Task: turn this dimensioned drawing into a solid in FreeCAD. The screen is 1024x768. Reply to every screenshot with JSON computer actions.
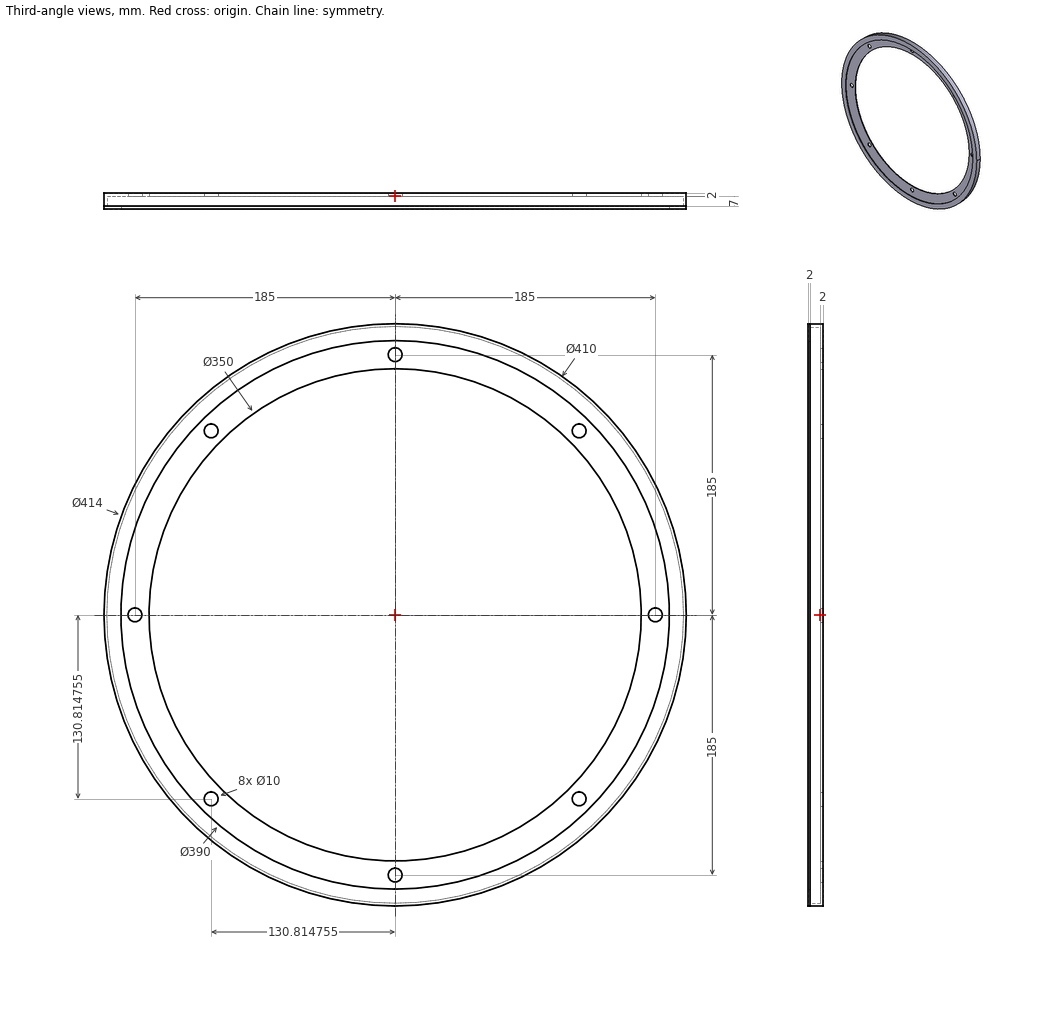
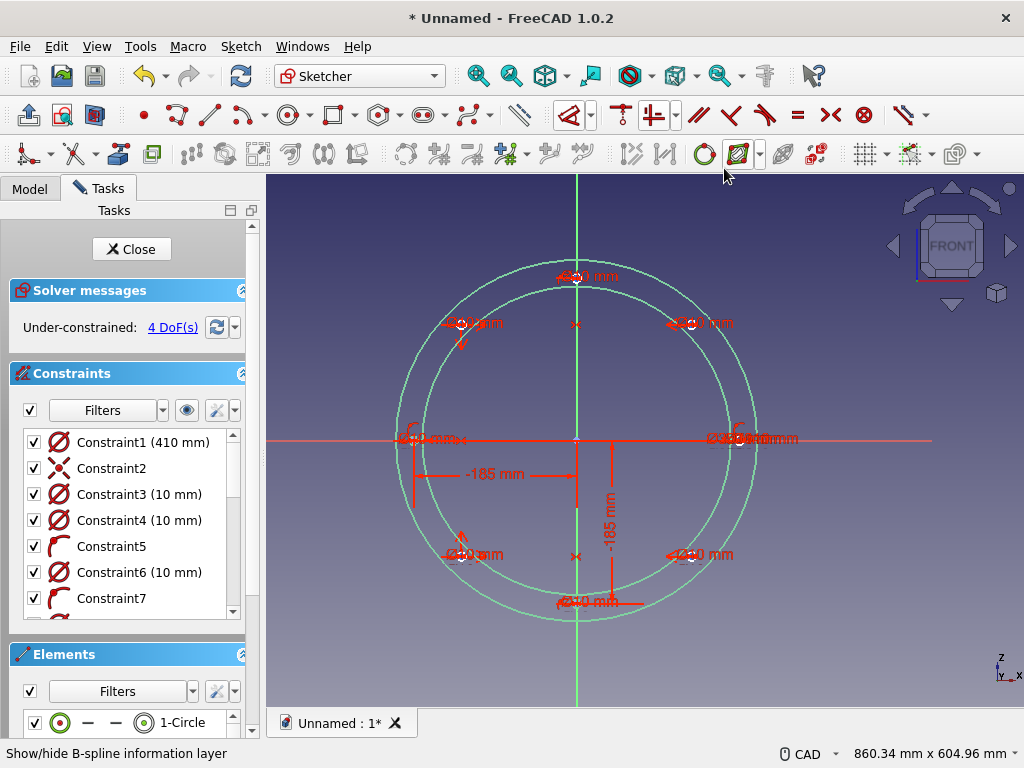
{"action": "left_click", "coordinate": [740, 441]}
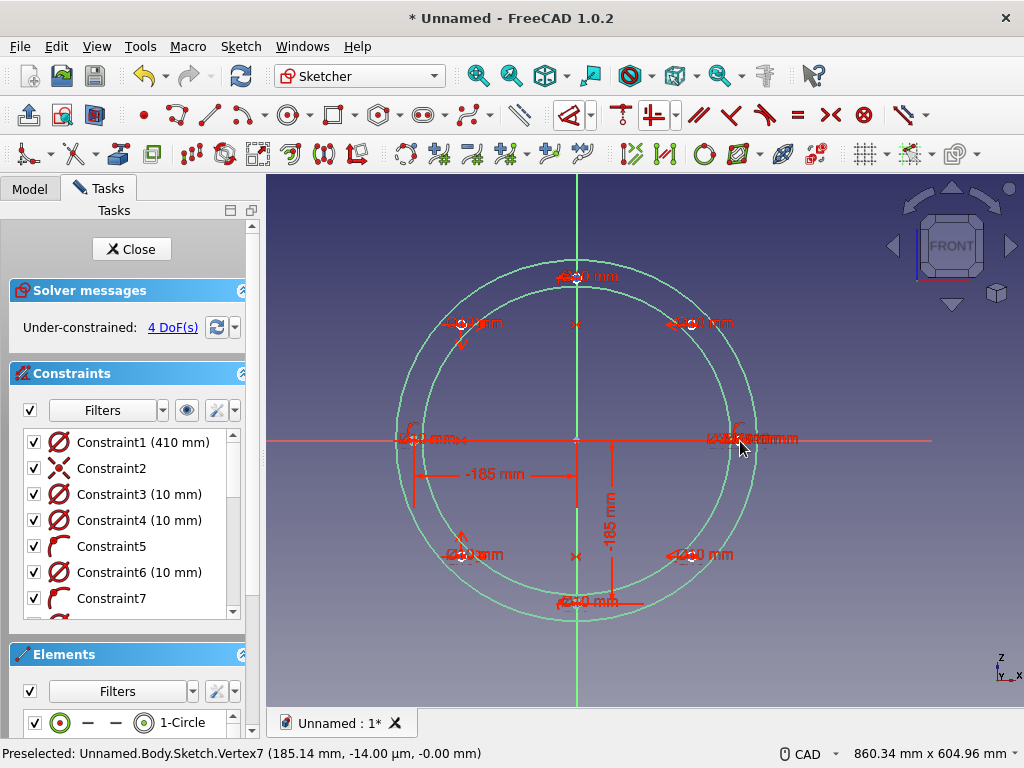
{"action": "left_click", "coordinate": [590, 116]}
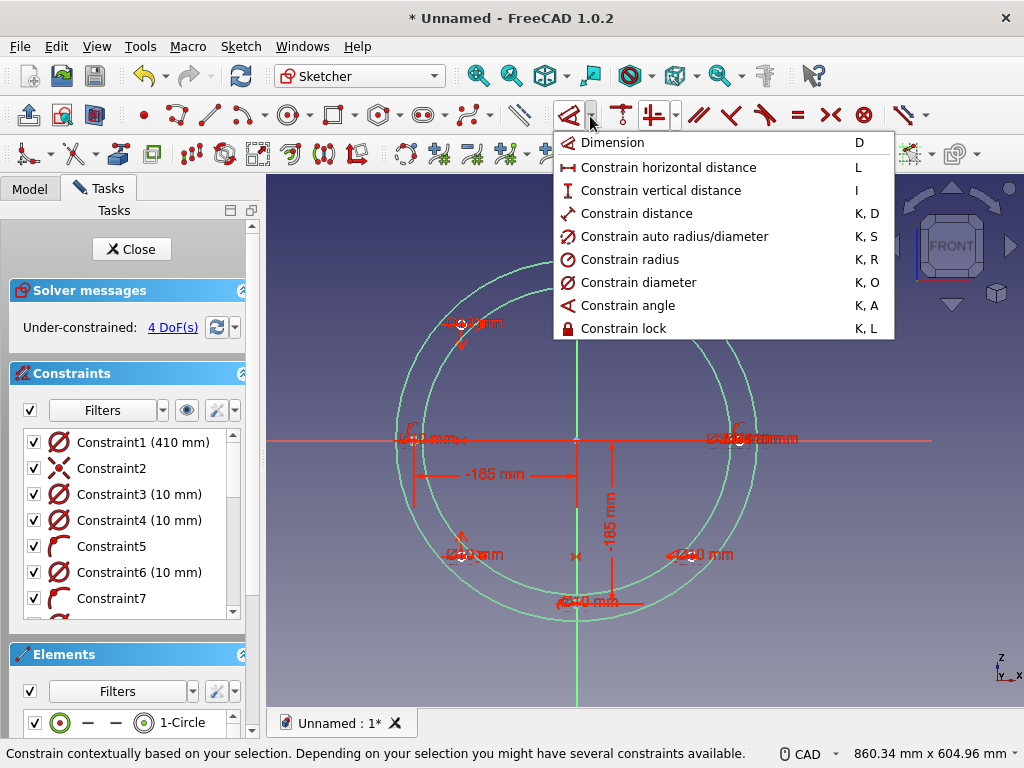
{"action": "left_click", "coordinate": [724, 168]}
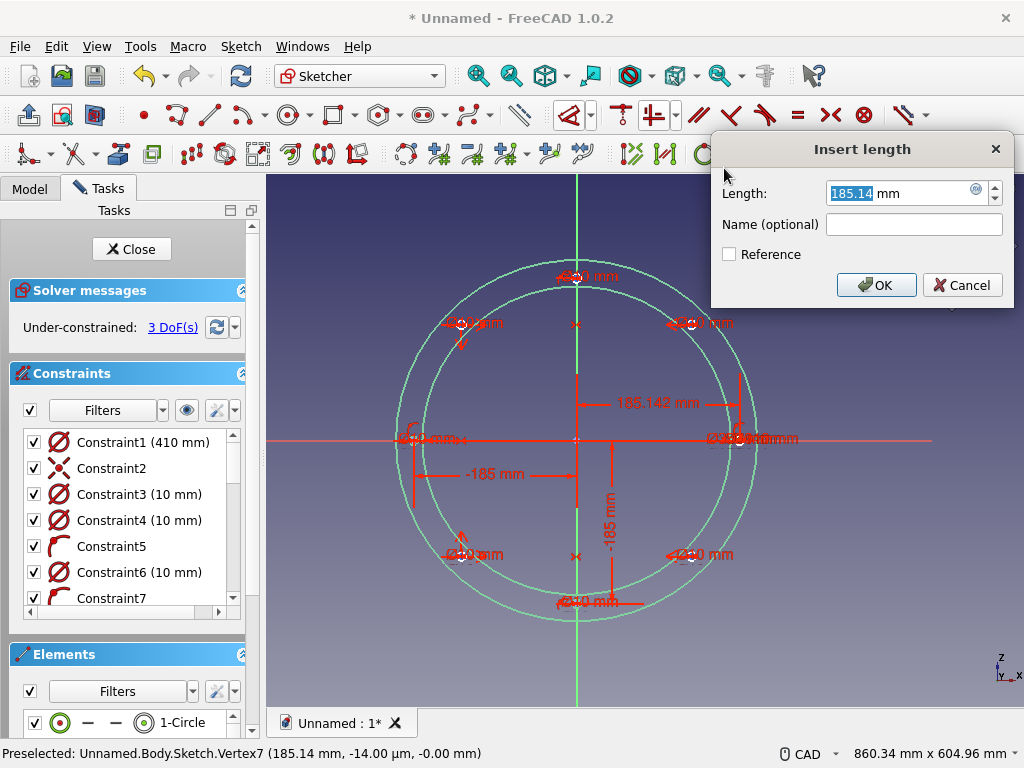
{"action": "type", "text": "185"}
{"action": "key", "text": "Return"}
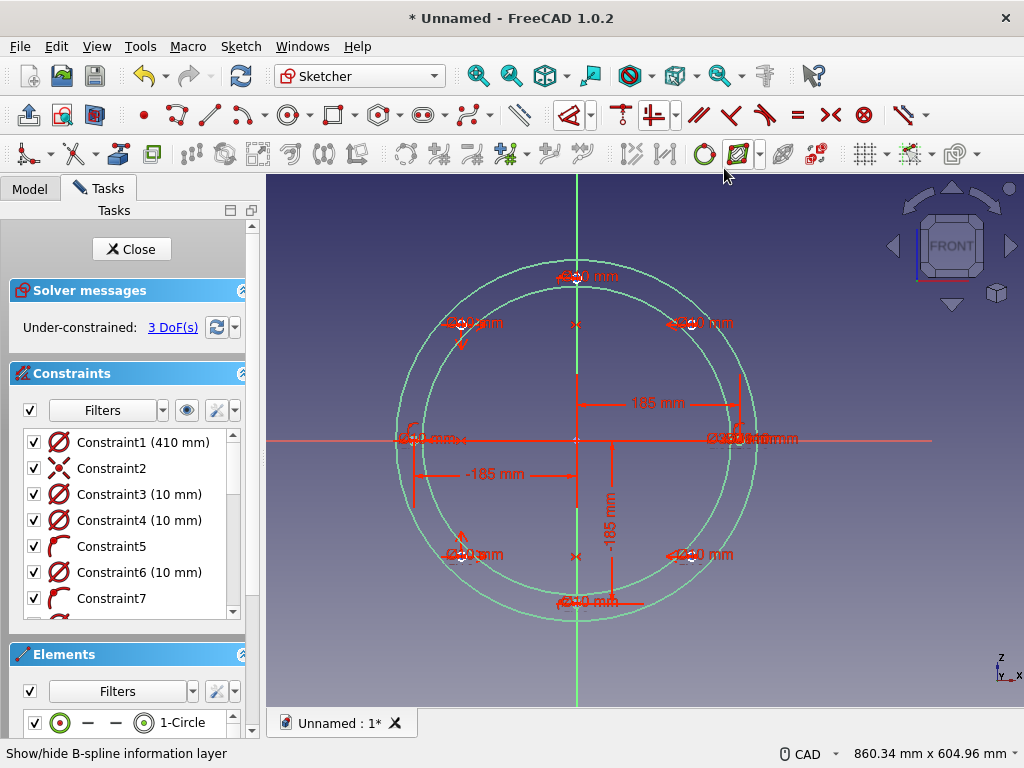
{"action": "left_click", "coordinate": [577, 278]}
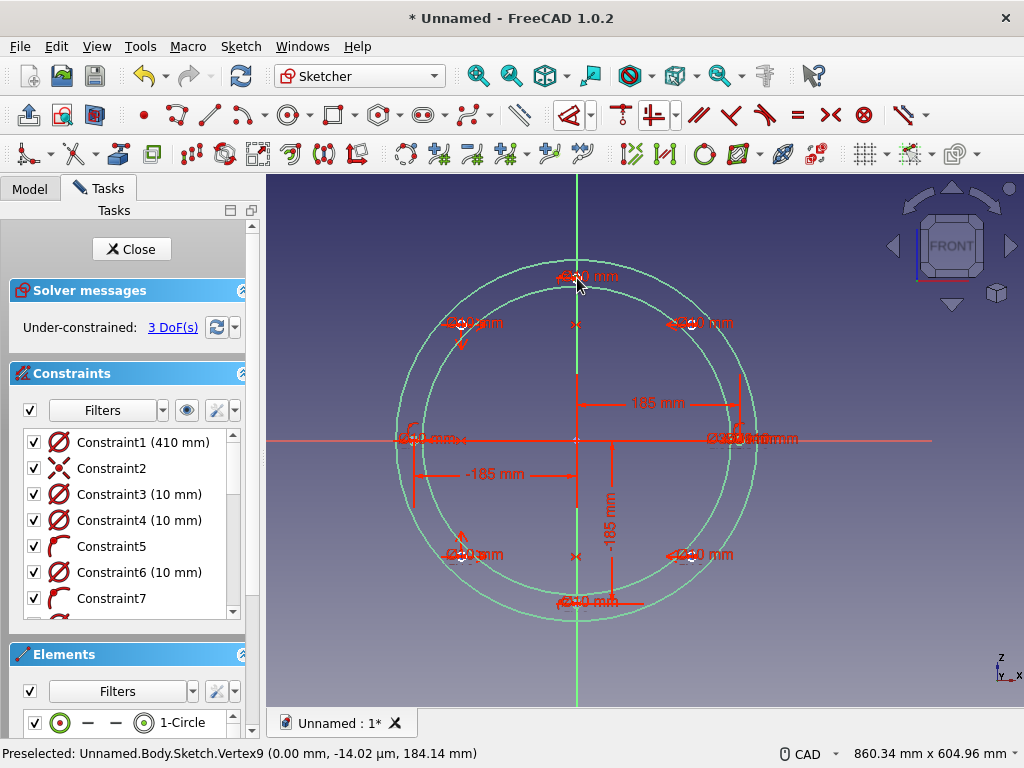
{"action": "key", "text": "i"}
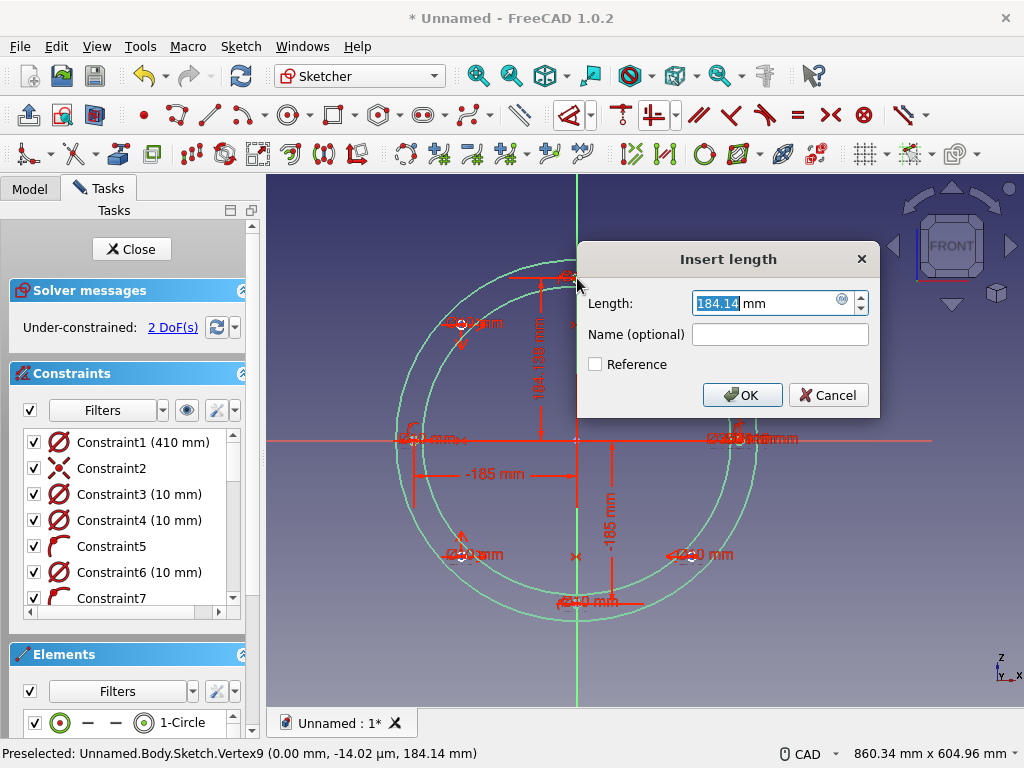
{"action": "type", "text": "185"}
{"action": "key", "text": "Return"}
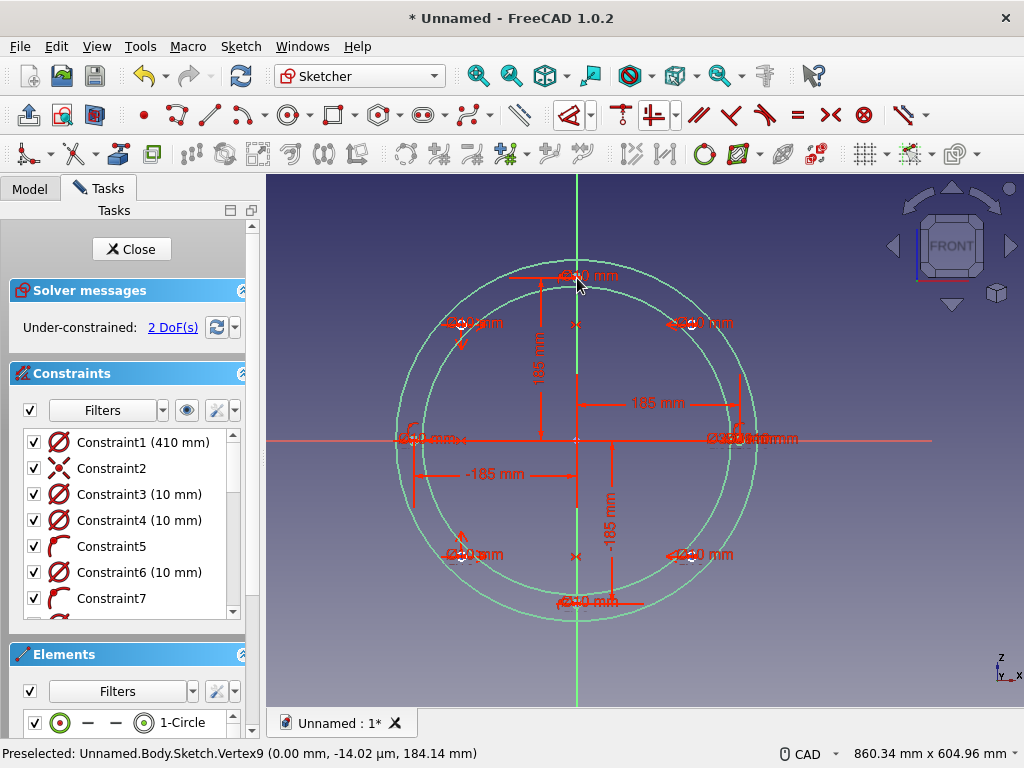
{"action": "left_click", "coordinate": [461, 557]}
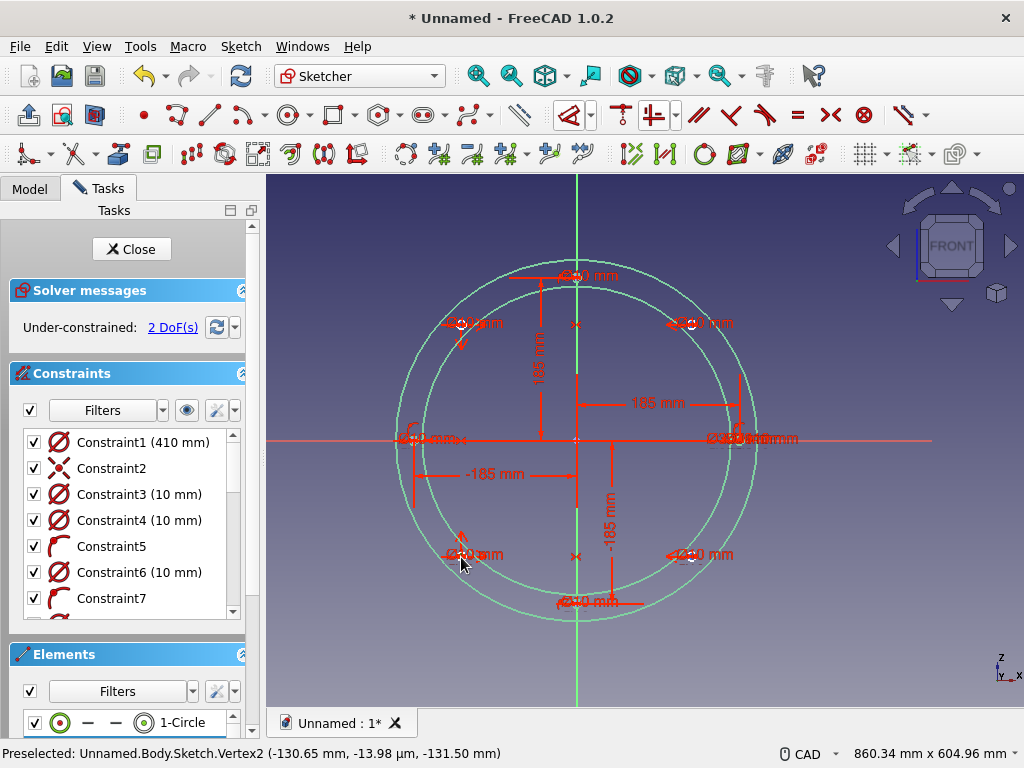
{"action": "key", "text": "l"}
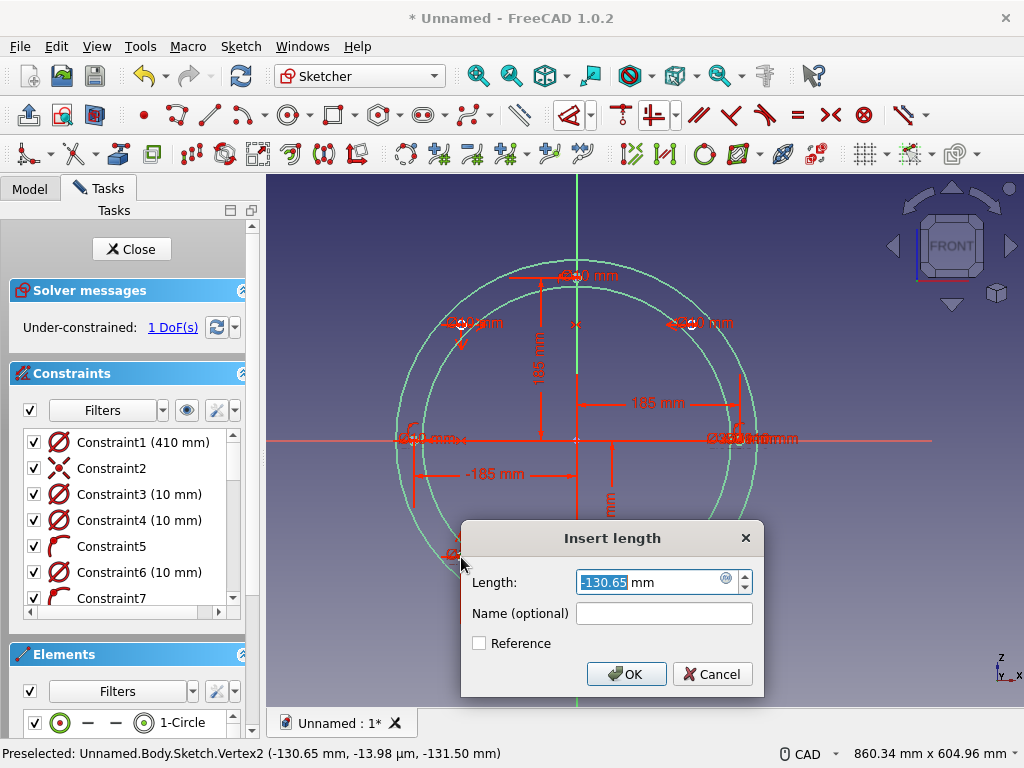
{"action": "type", "text": "-130.814755"}
{"action": "key", "text": "Return"}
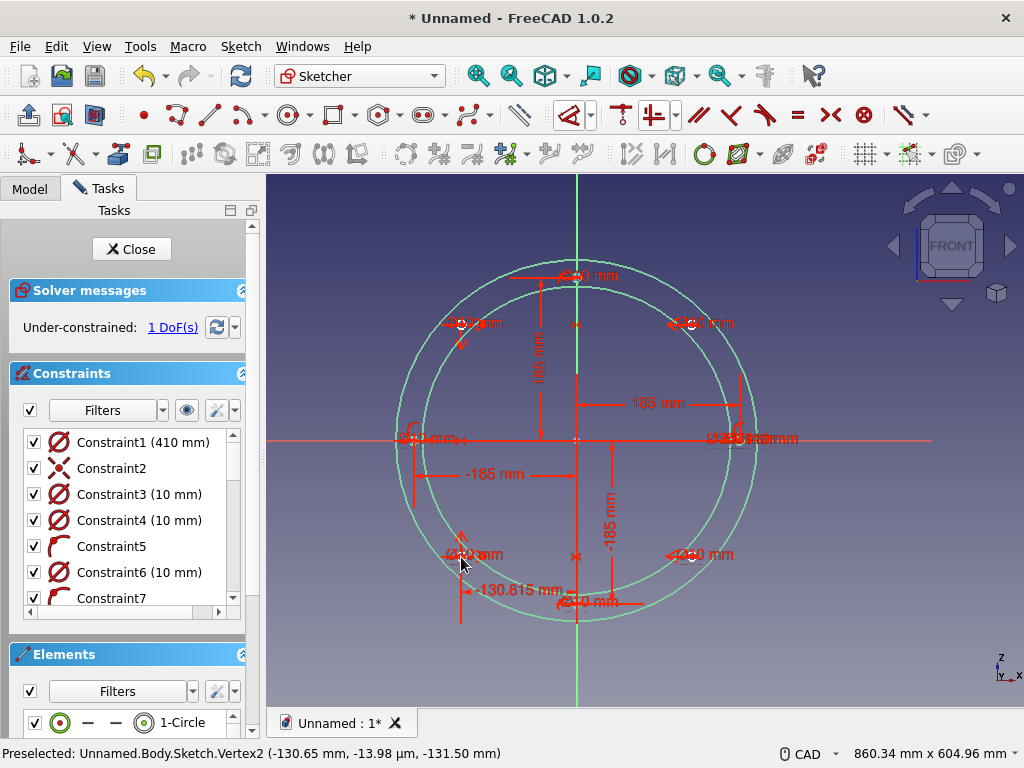
{"action": "left_click", "coordinate": [461, 557]}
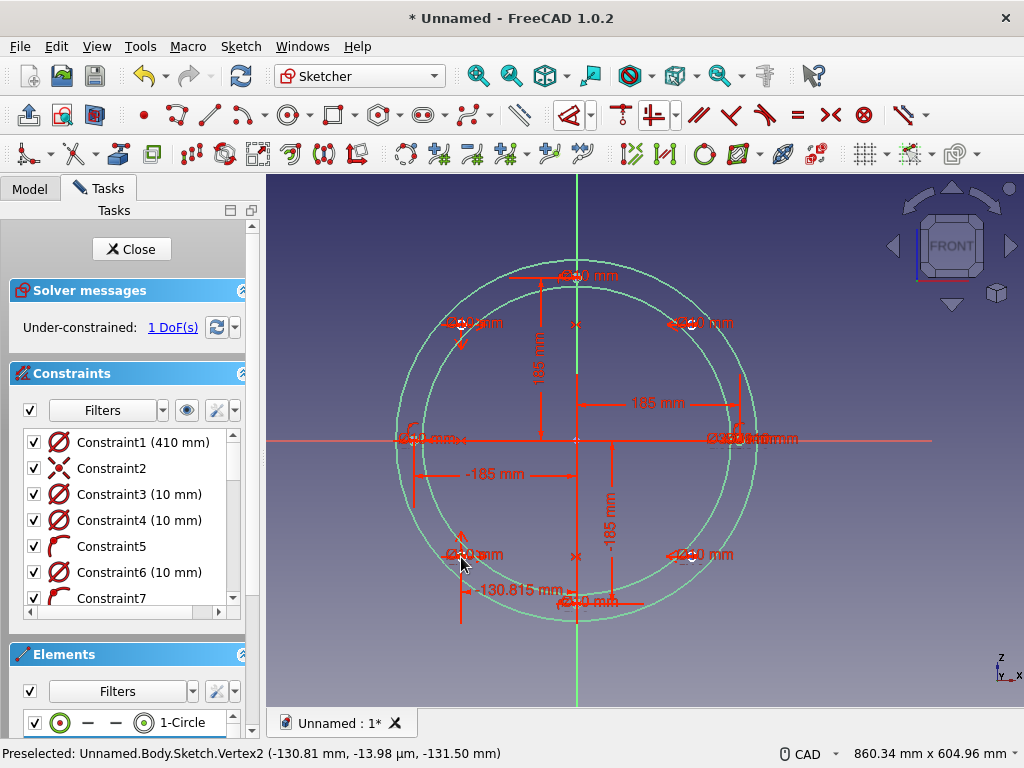
{"action": "left_click", "coordinate": [590, 116]}